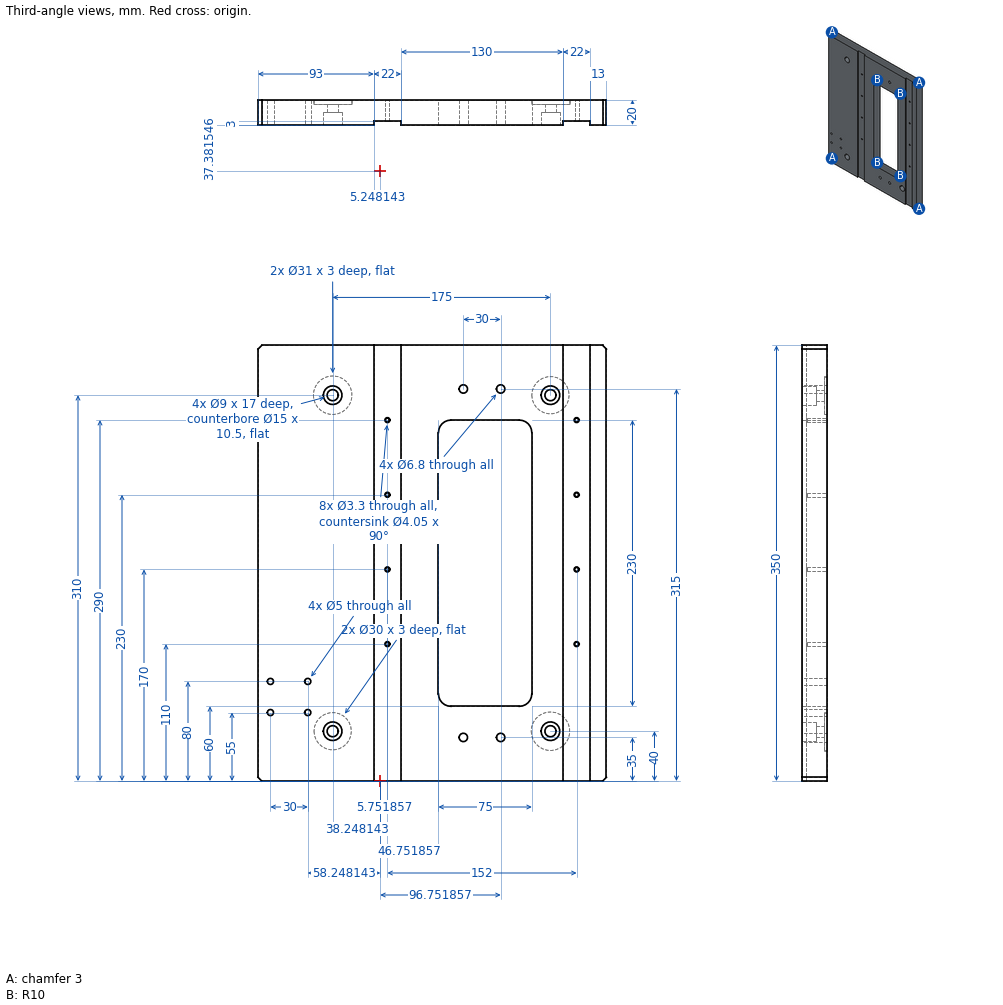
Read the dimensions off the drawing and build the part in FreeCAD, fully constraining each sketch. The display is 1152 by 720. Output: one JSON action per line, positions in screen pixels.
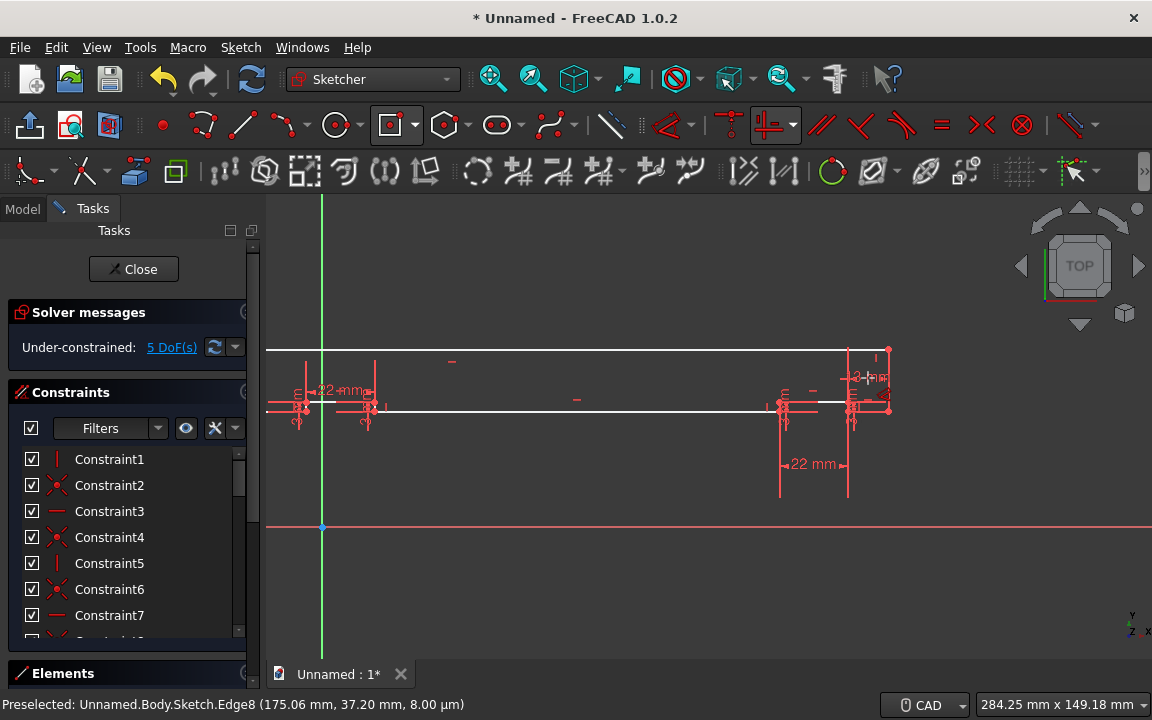
{"action": "left_click", "coordinate": [889, 393]}
{"action": "left_click", "coordinate": [947, 381]}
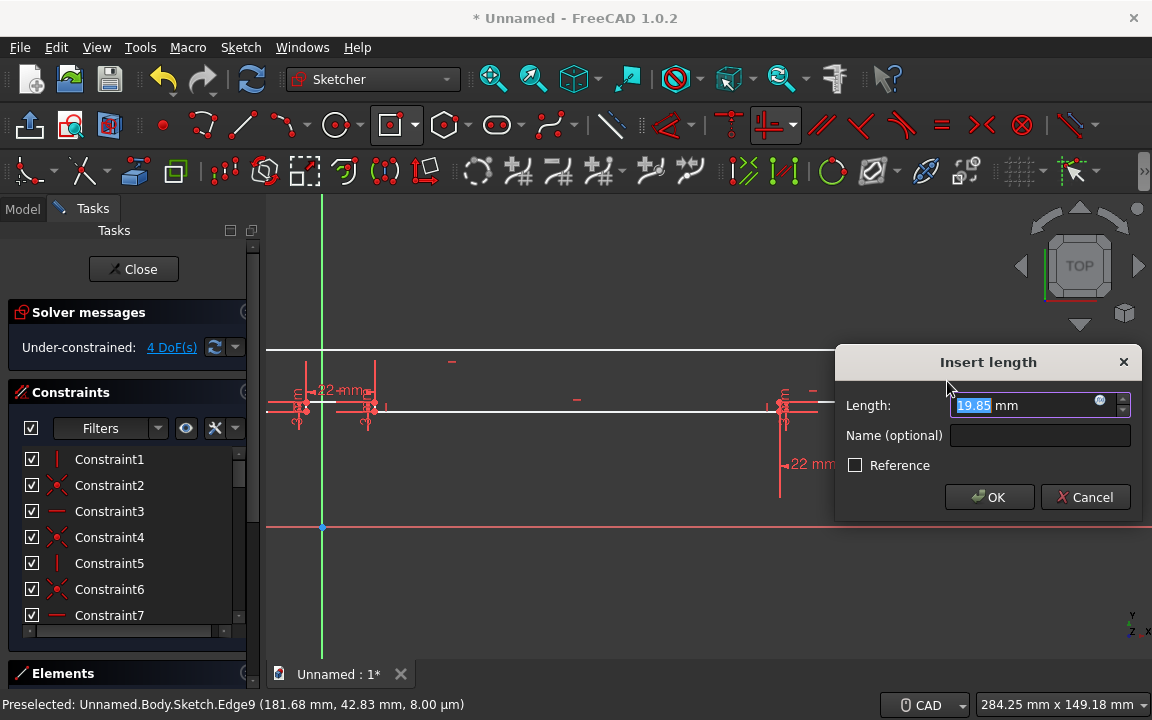
{"action": "type", "text": "20"}
{"action": "key", "text": "Return"}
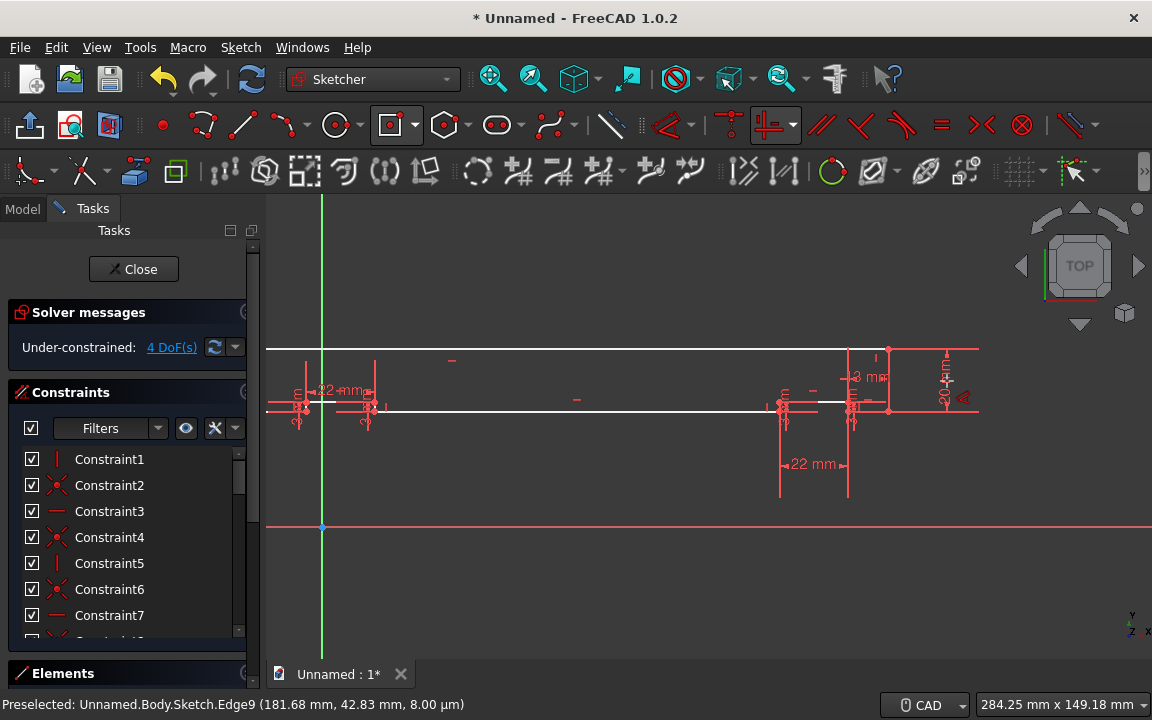
{"action": "scroll", "coordinate": [869, 412], "scroll_direction": "down", "scroll_amount": 3}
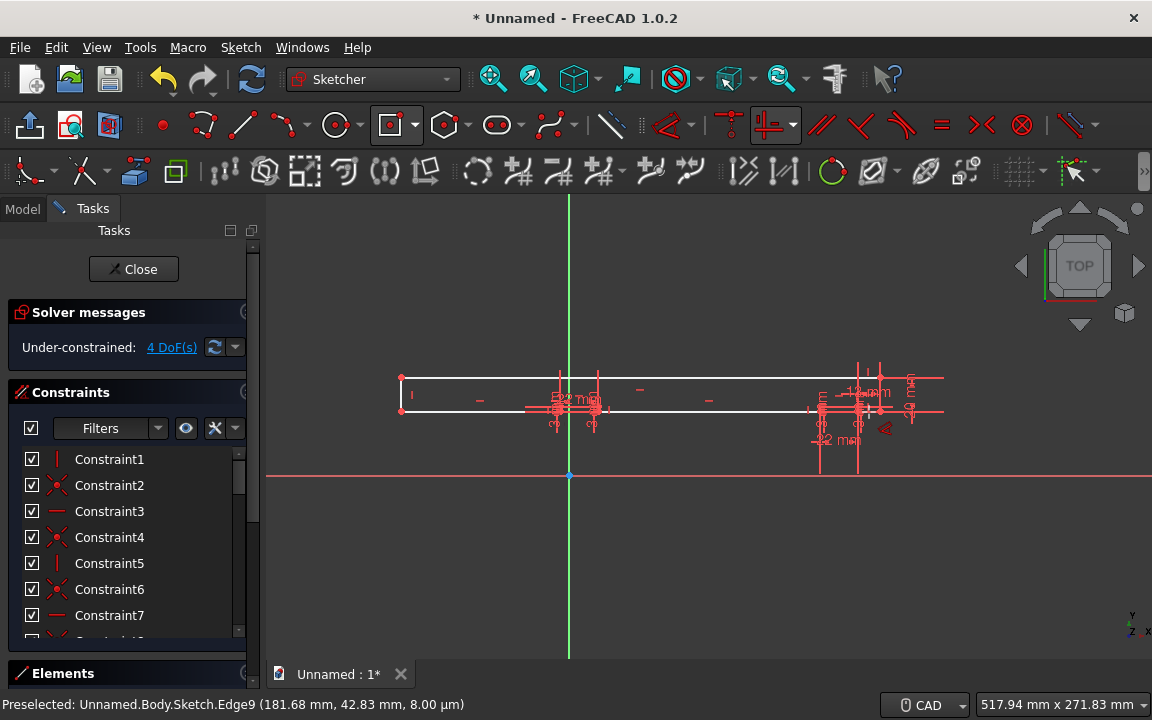
{"action": "left_click", "coordinate": [449, 412]}
{"action": "left_click", "coordinate": [481, 446]}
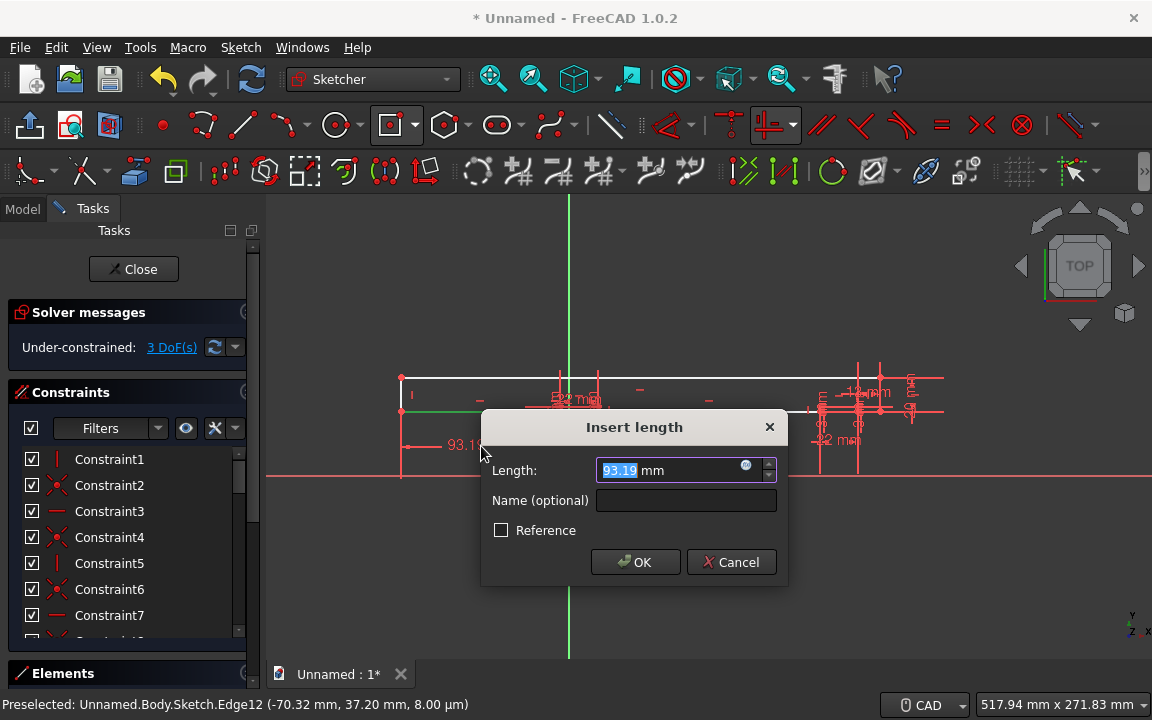
{"action": "type", "text": "93"}
{"action": "key", "text": "Return"}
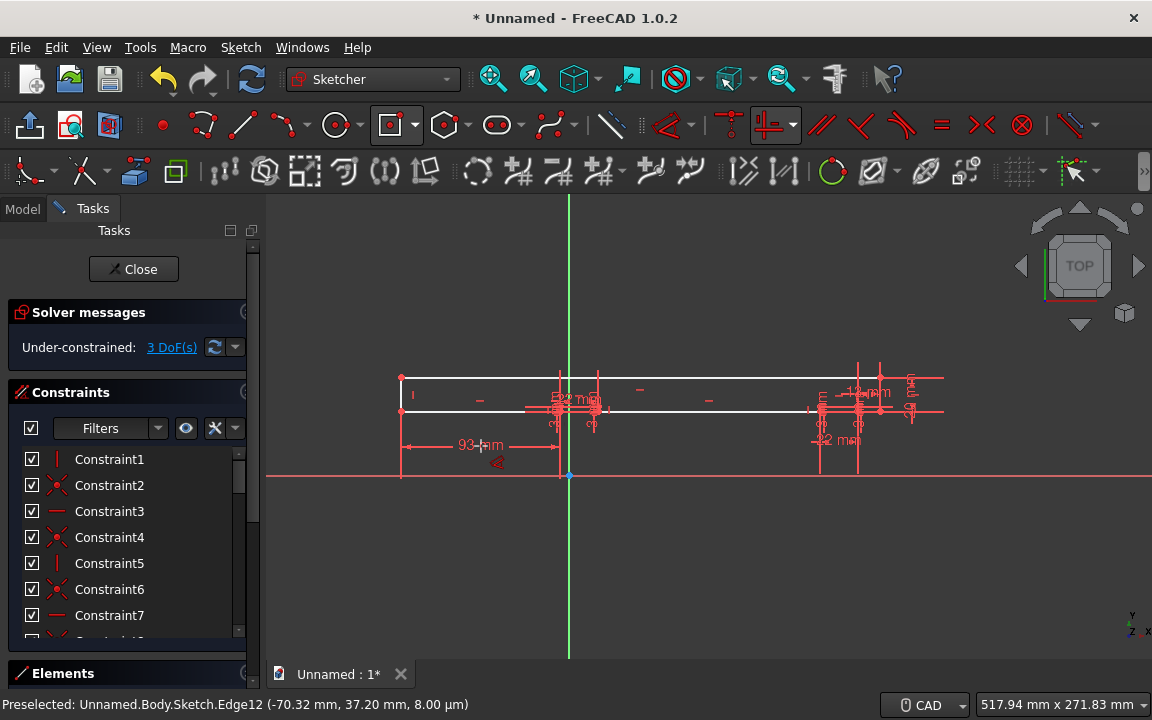
{"action": "left_click", "coordinate": [665, 412]}
{"action": "left_click", "coordinate": [709, 446]}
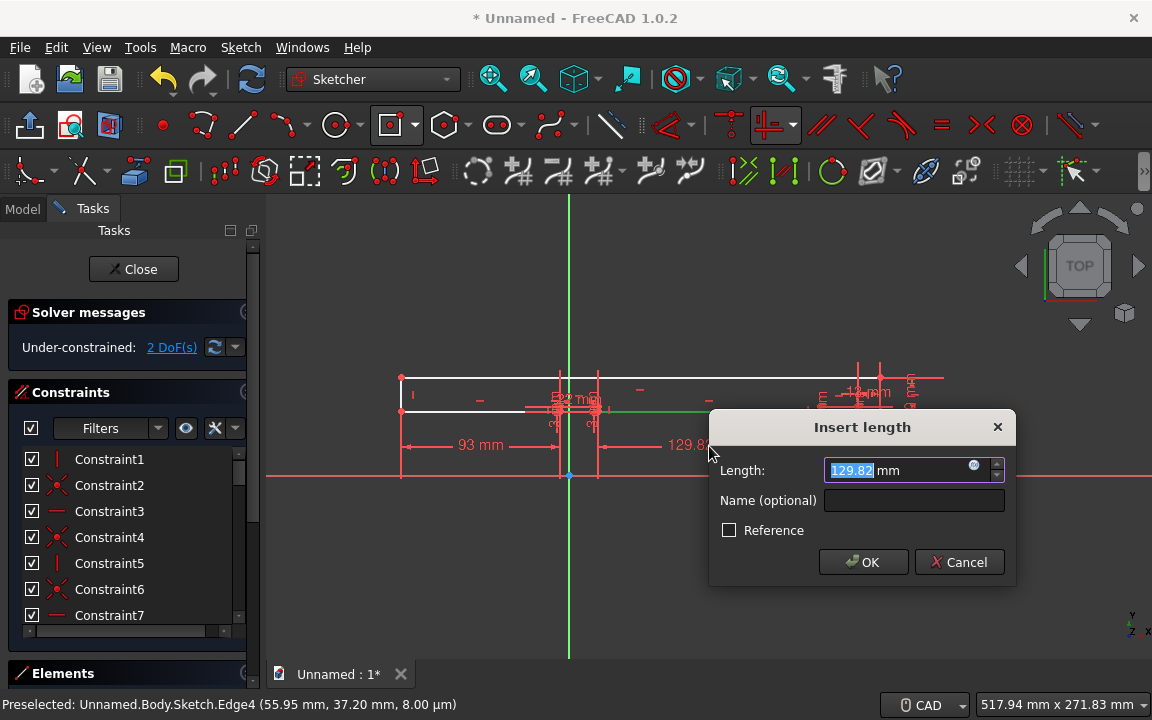
{"action": "type", "text": "130"}
{"action": "key", "text": "Return"}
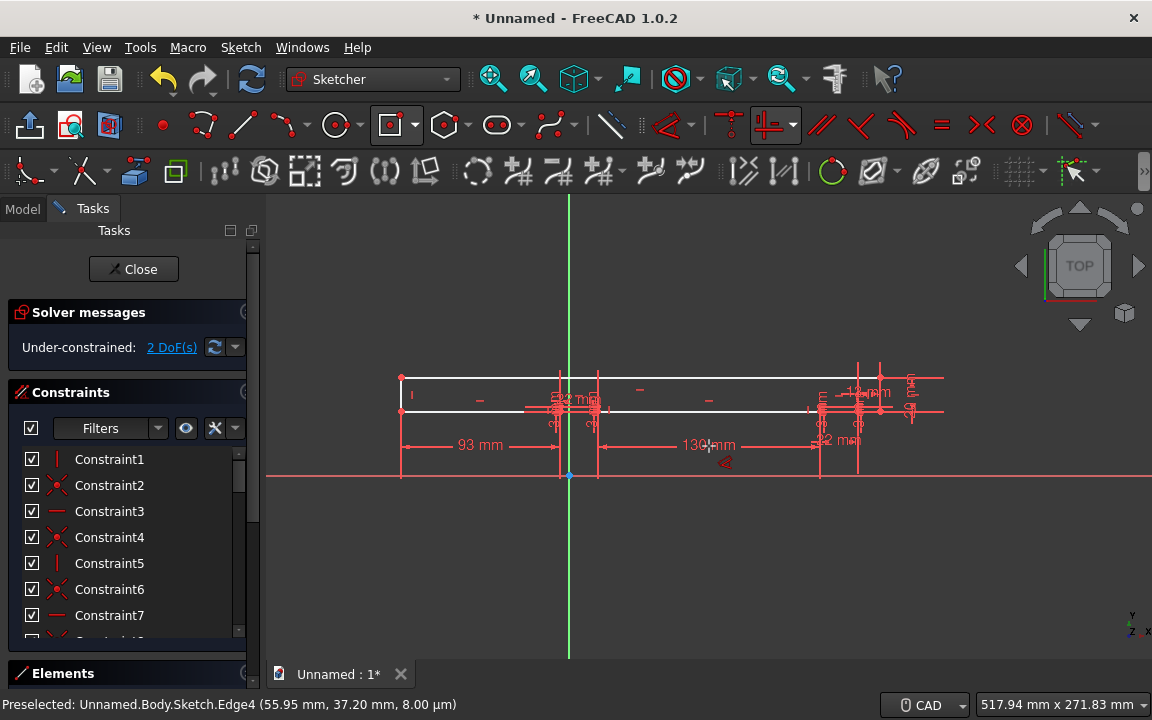
{"action": "scroll", "coordinate": [560, 412], "scroll_direction": "up", "scroll_amount": 8}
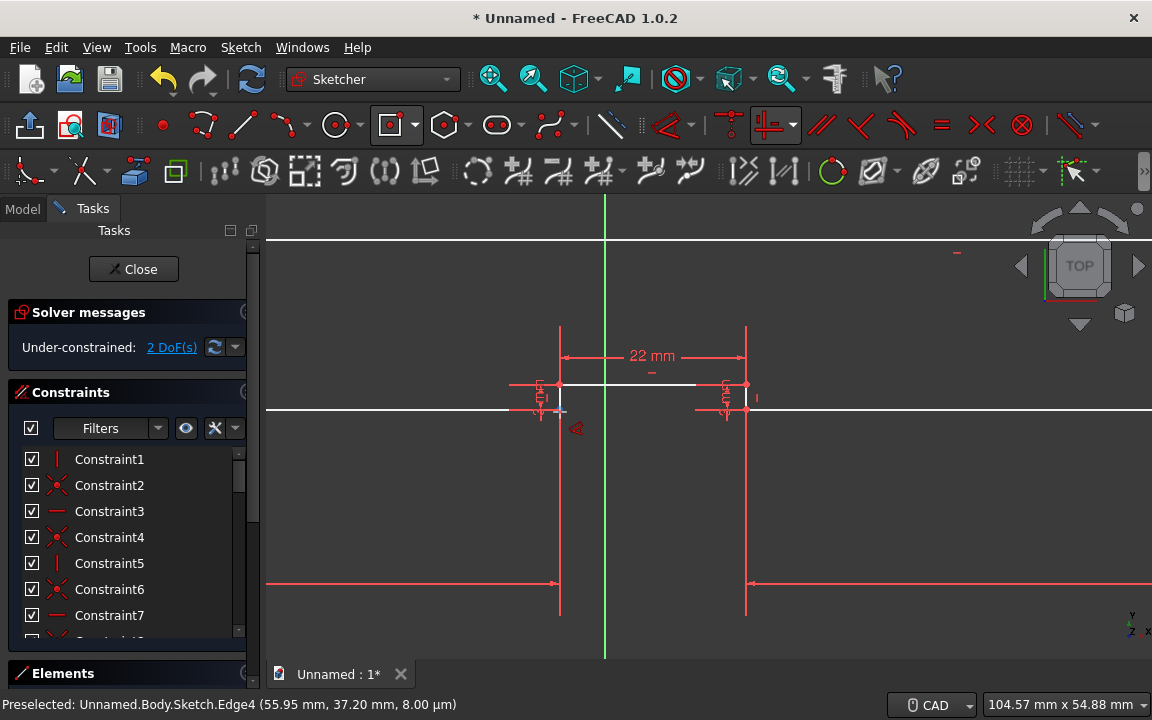
{"action": "left_click", "coordinate": [560, 410]}
{"action": "left_click", "coordinate": [582, 352]}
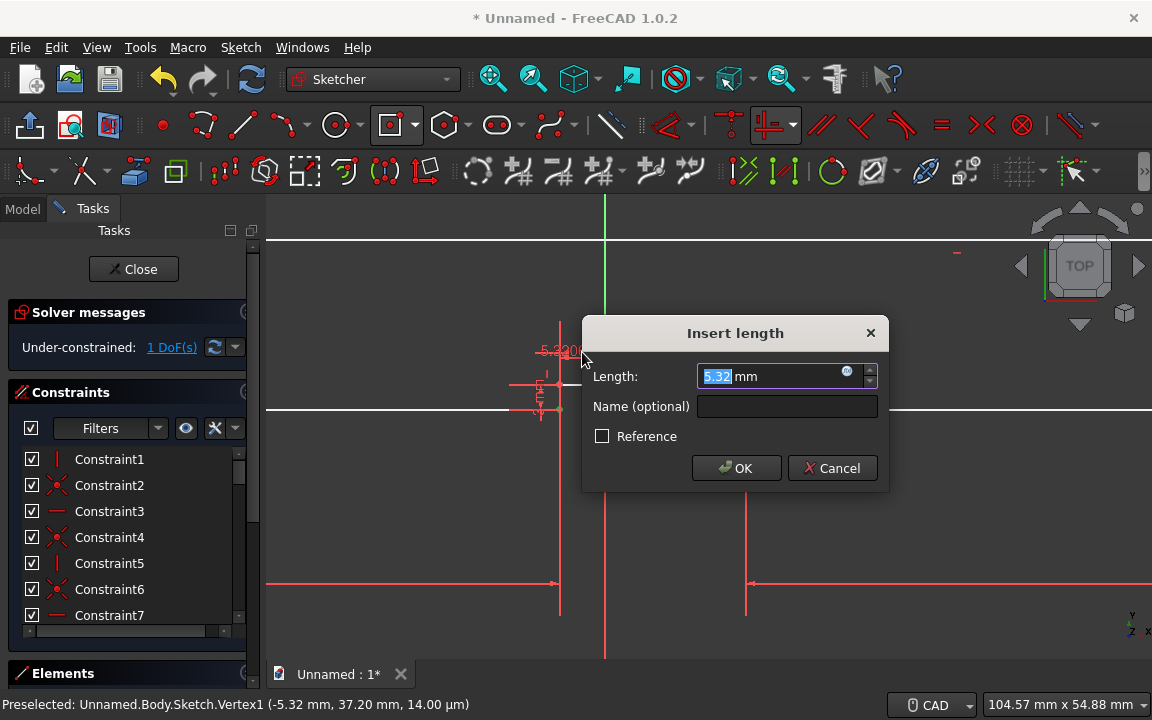
{"action": "type", "text": "5.248143"}
{"action": "key", "text": "Return"}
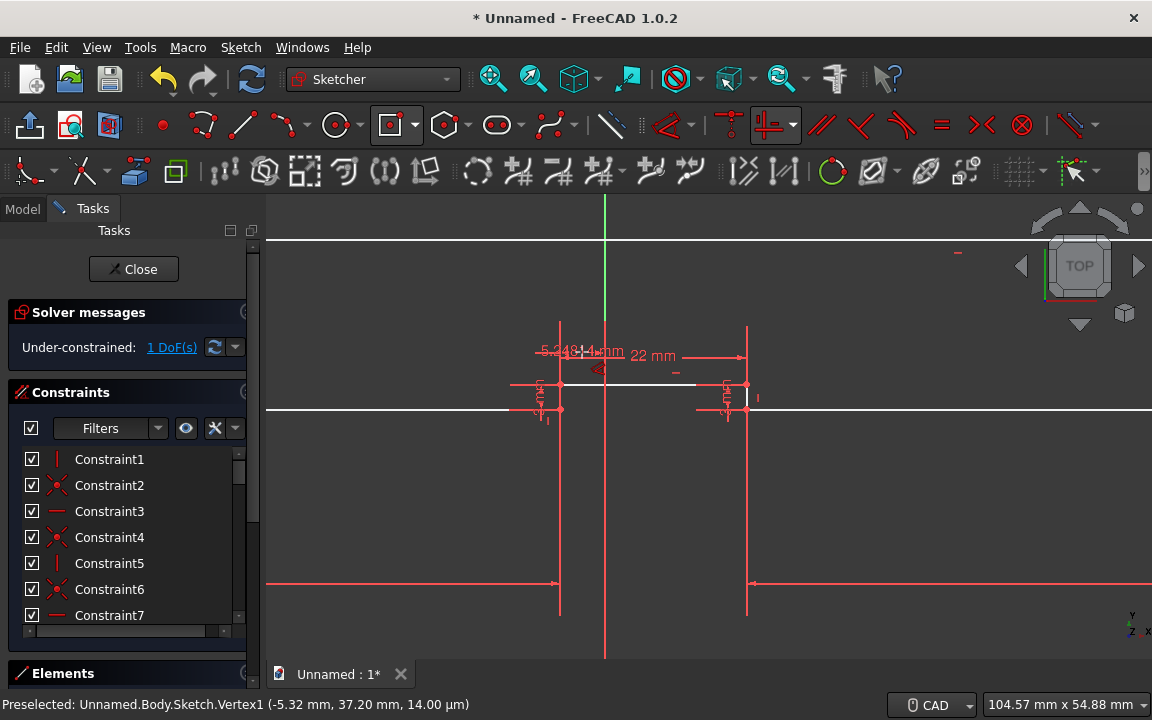
{"action": "left_click", "coordinate": [560, 410]}
{"action": "left_click", "coordinate": [526, 520]}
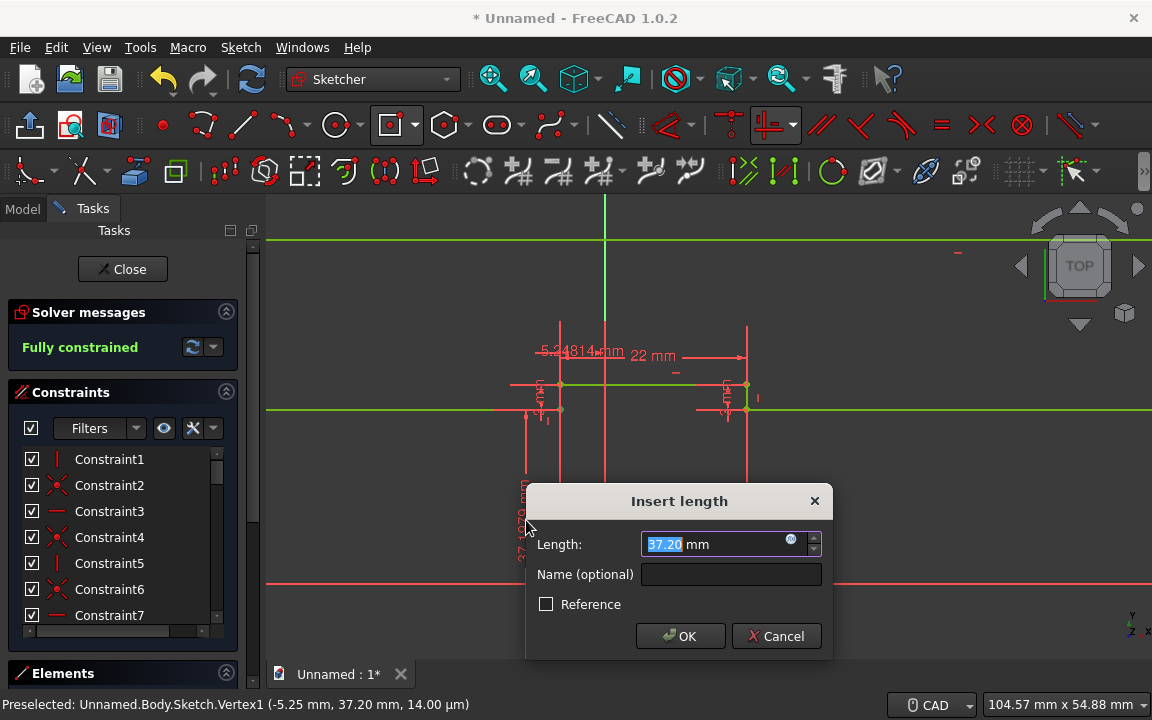
{"action": "type", "text": "37.381546"}
{"action": "key", "text": "Return"}
{"action": "key", "text": "Escape"}